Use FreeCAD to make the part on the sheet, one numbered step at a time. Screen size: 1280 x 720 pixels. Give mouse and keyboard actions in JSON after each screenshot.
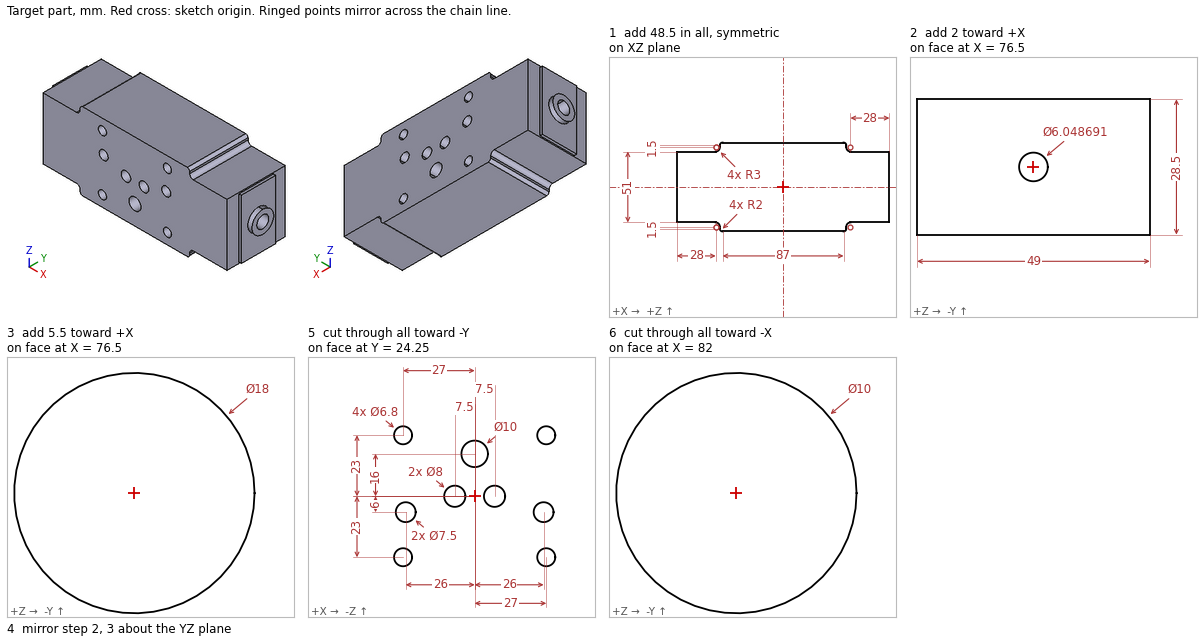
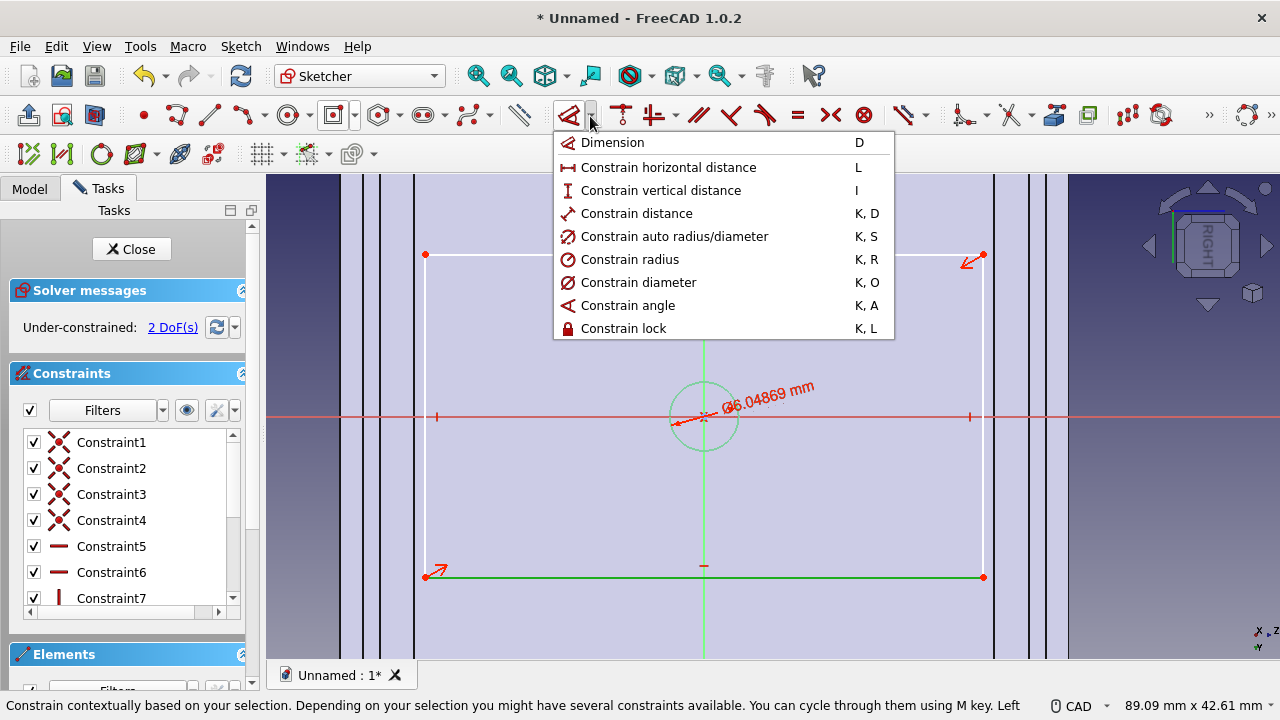
{"action": "left_click", "coordinate": [724, 168]}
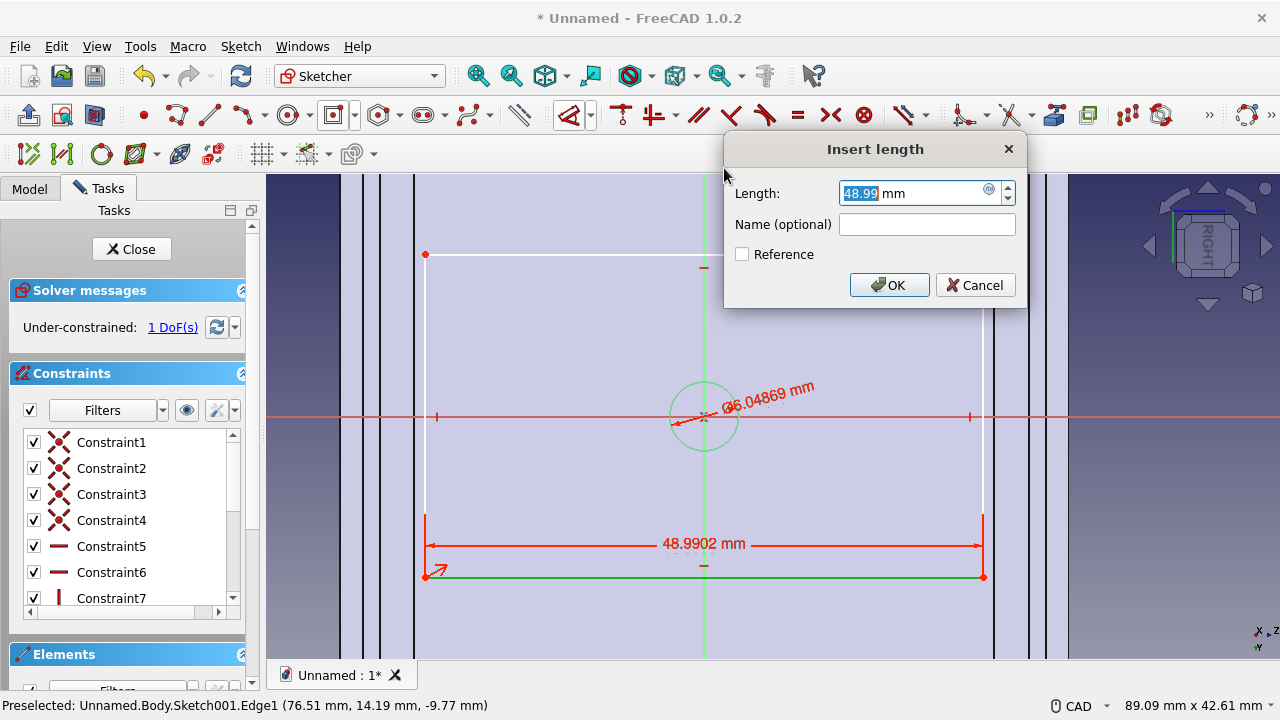
{"action": "type", "text": "49"}
{"action": "key", "text": "Return"}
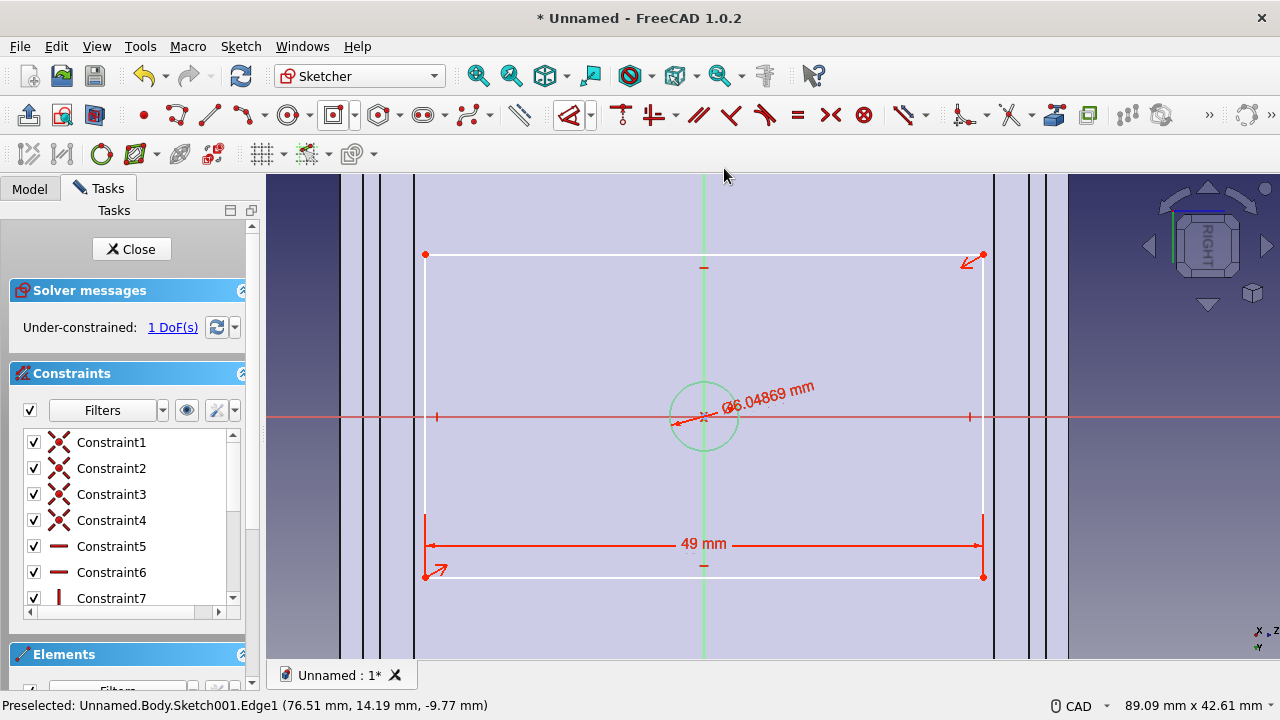
{"action": "left_click", "coordinate": [983, 481]}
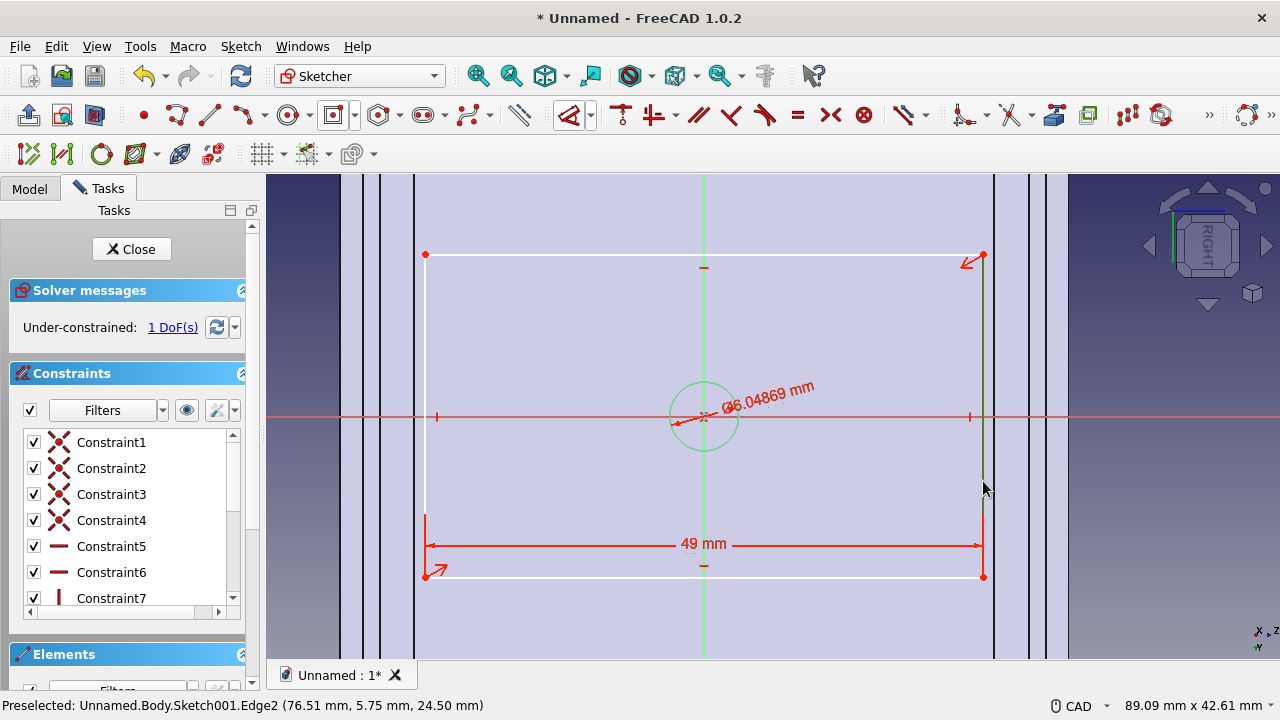
{"action": "key", "text": "i"}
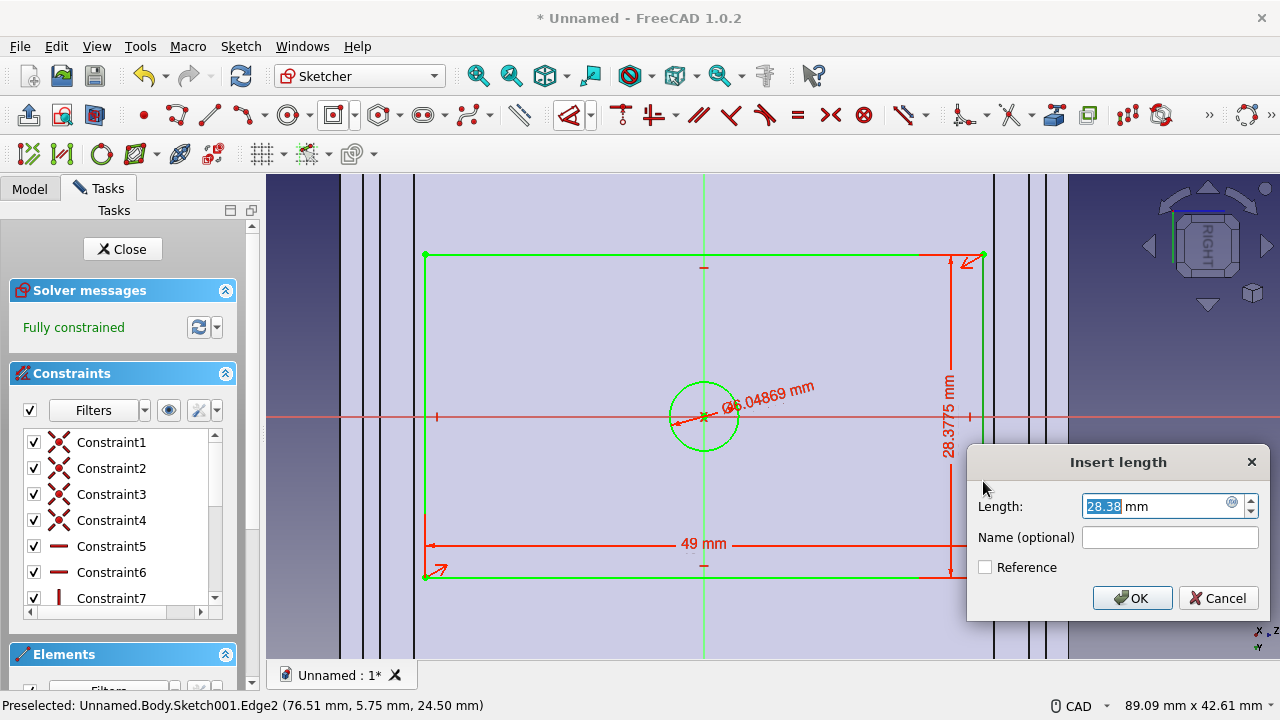
{"action": "type", "text": "28.5"}
{"action": "key", "text": "Return"}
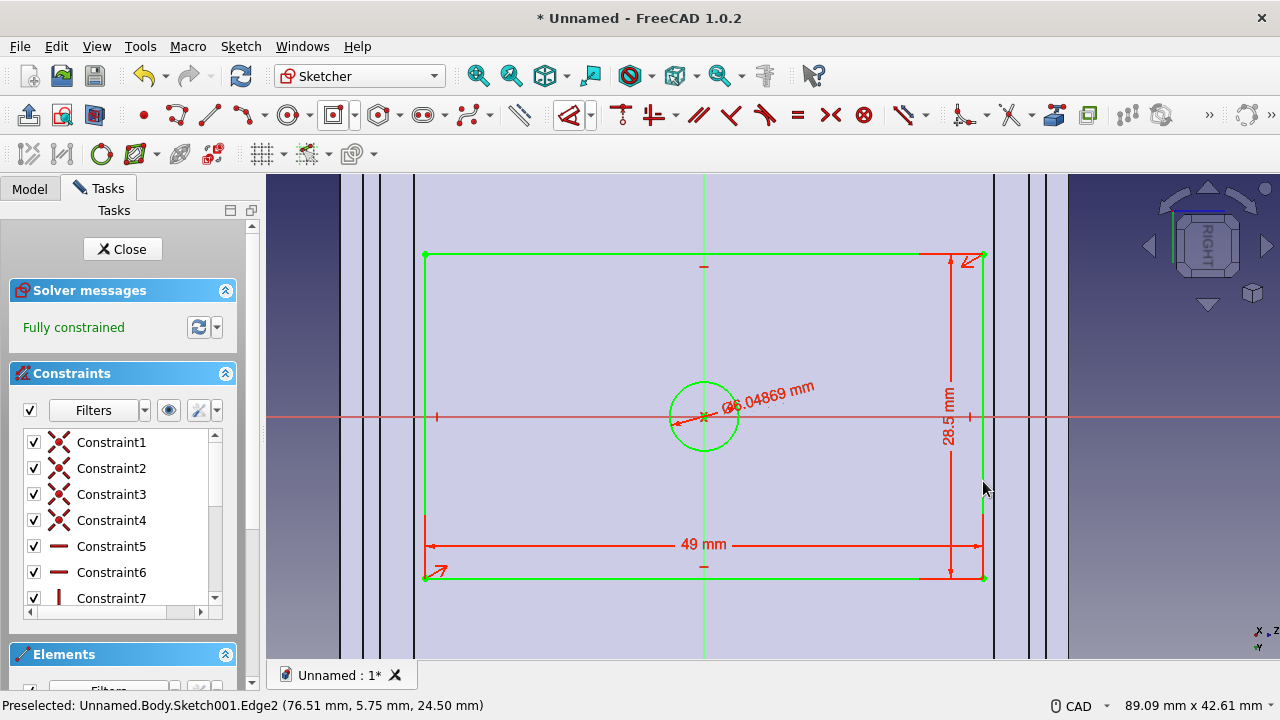
{"action": "left_click", "coordinate": [123, 249]}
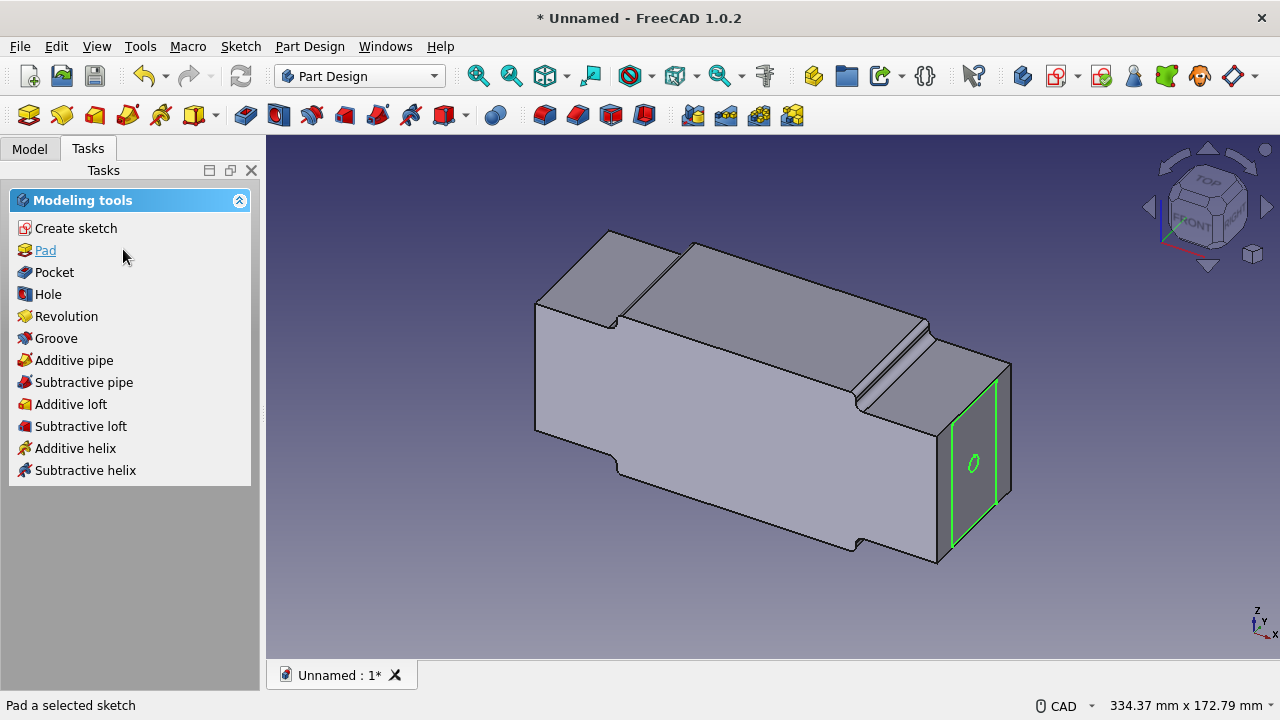
{"action": "left_click", "coordinate": [29, 116]}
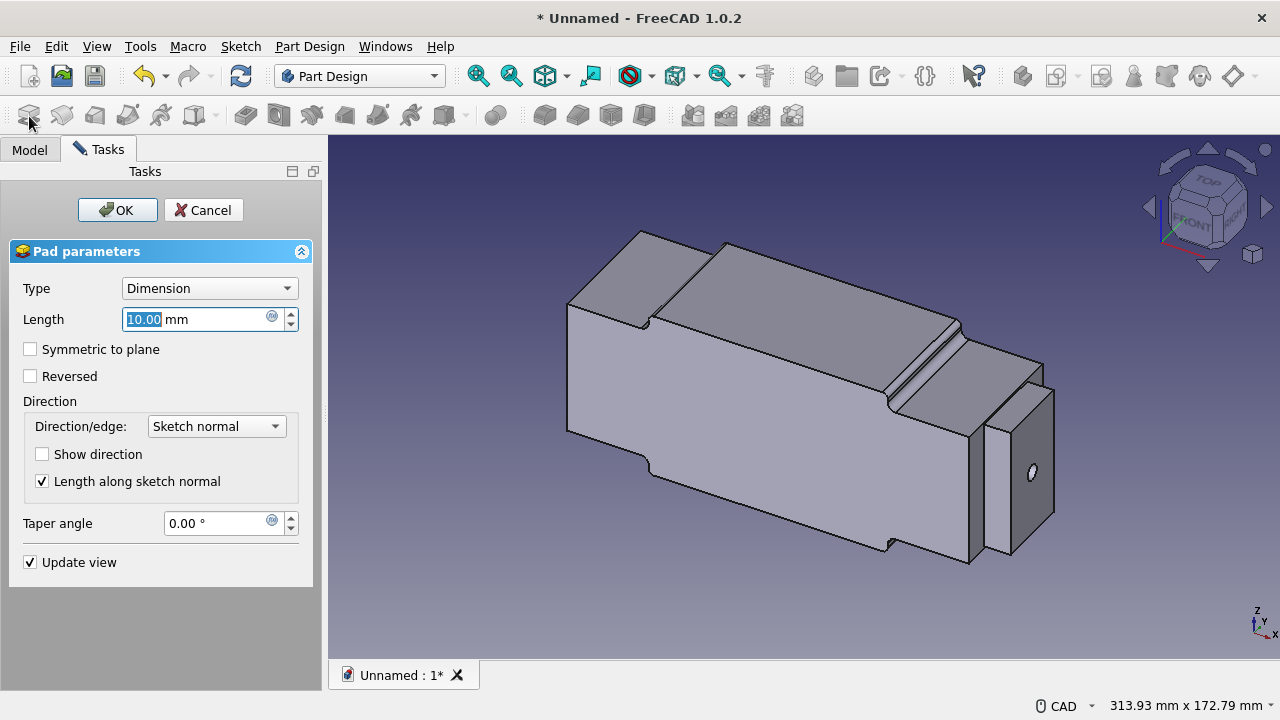
{"action": "type", "text": "2"}
{"action": "key", "text": "Tab"}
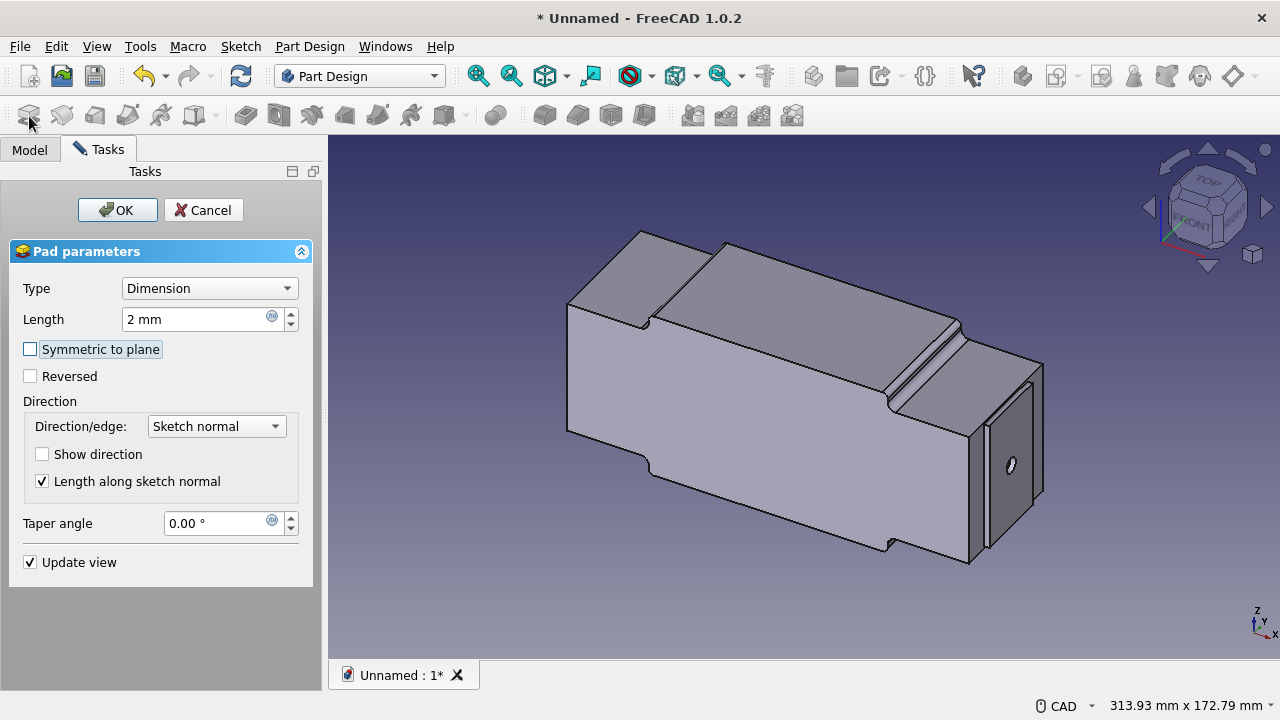
{"action": "left_click", "coordinate": [118, 210]}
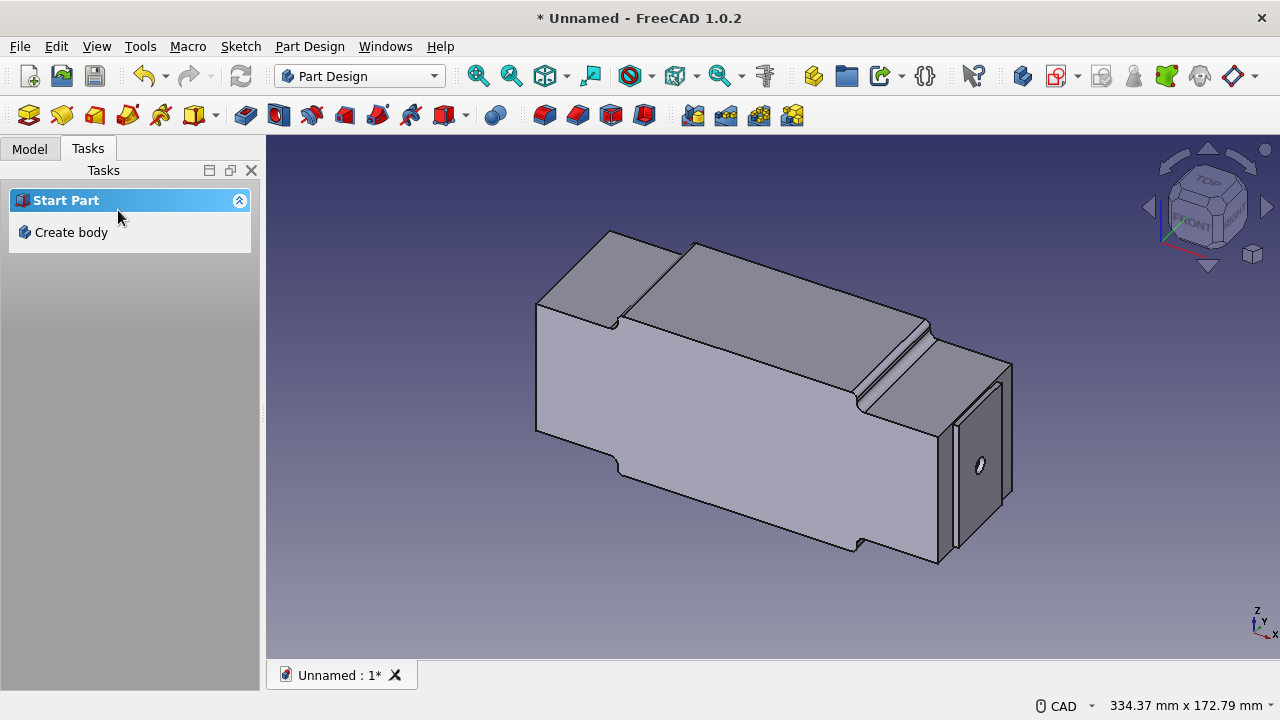
{"action": "key", "text": "0"}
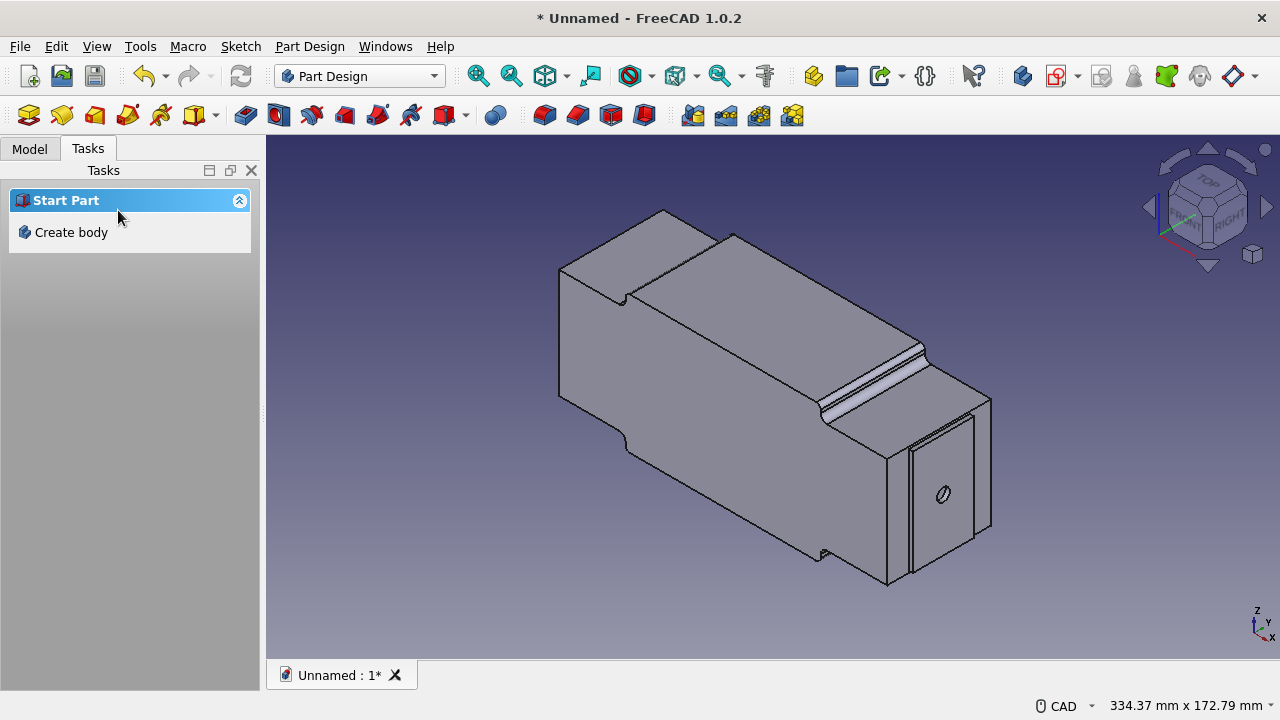
{"action": "left_click", "coordinate": [984, 484]}